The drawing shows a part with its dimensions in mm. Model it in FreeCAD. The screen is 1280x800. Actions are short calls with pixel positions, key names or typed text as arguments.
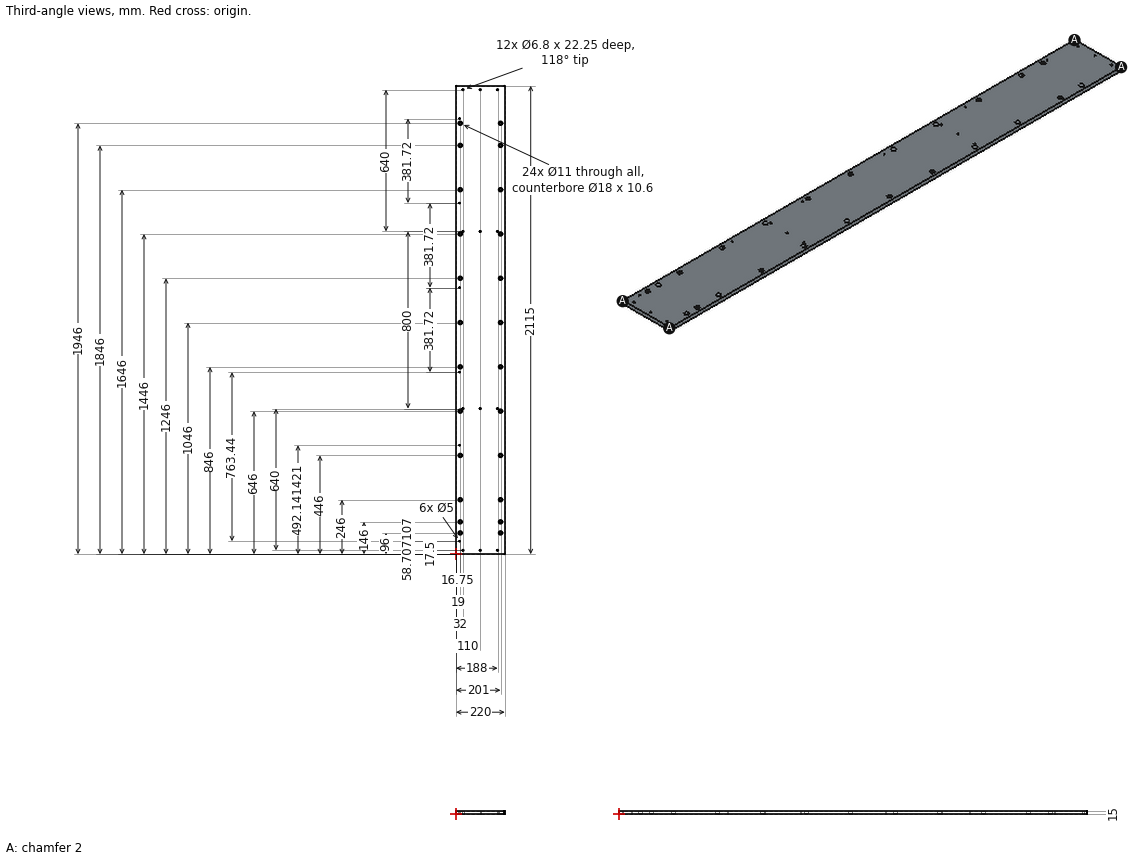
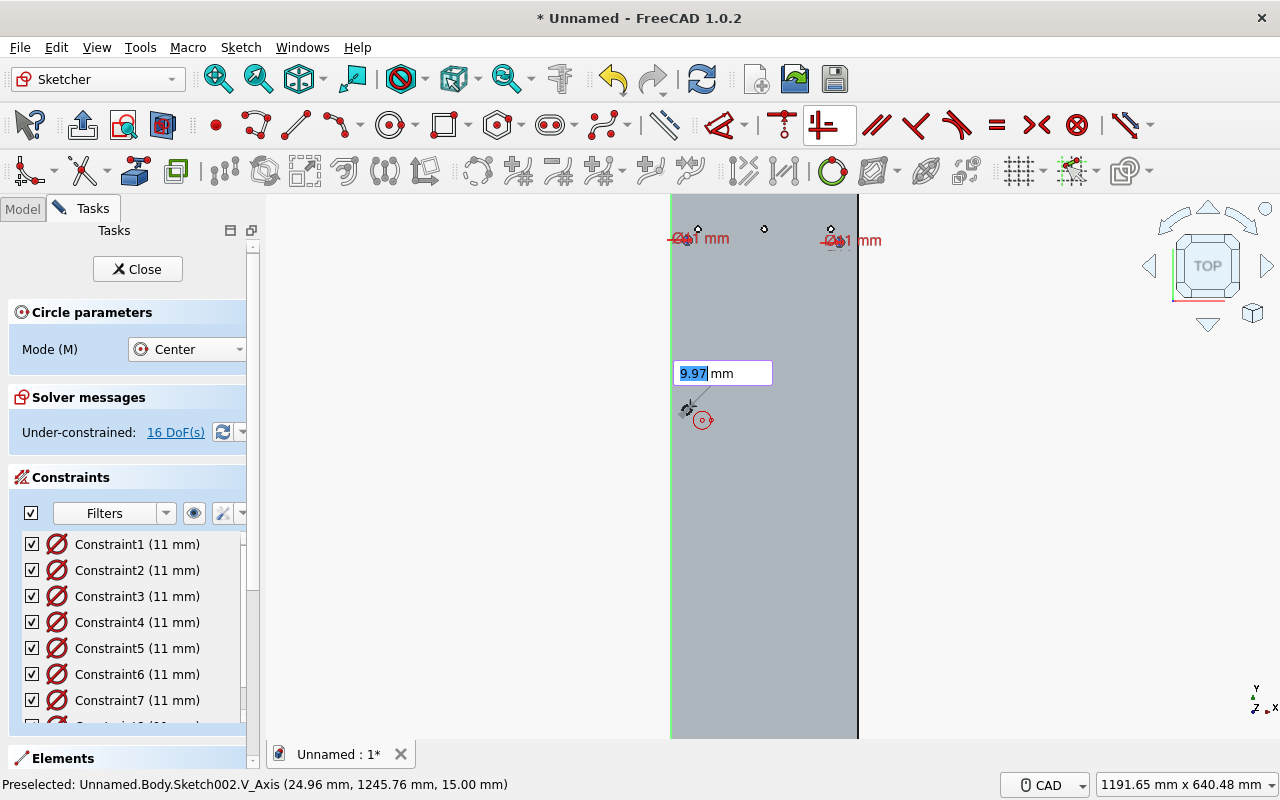
text(11)
key(Return)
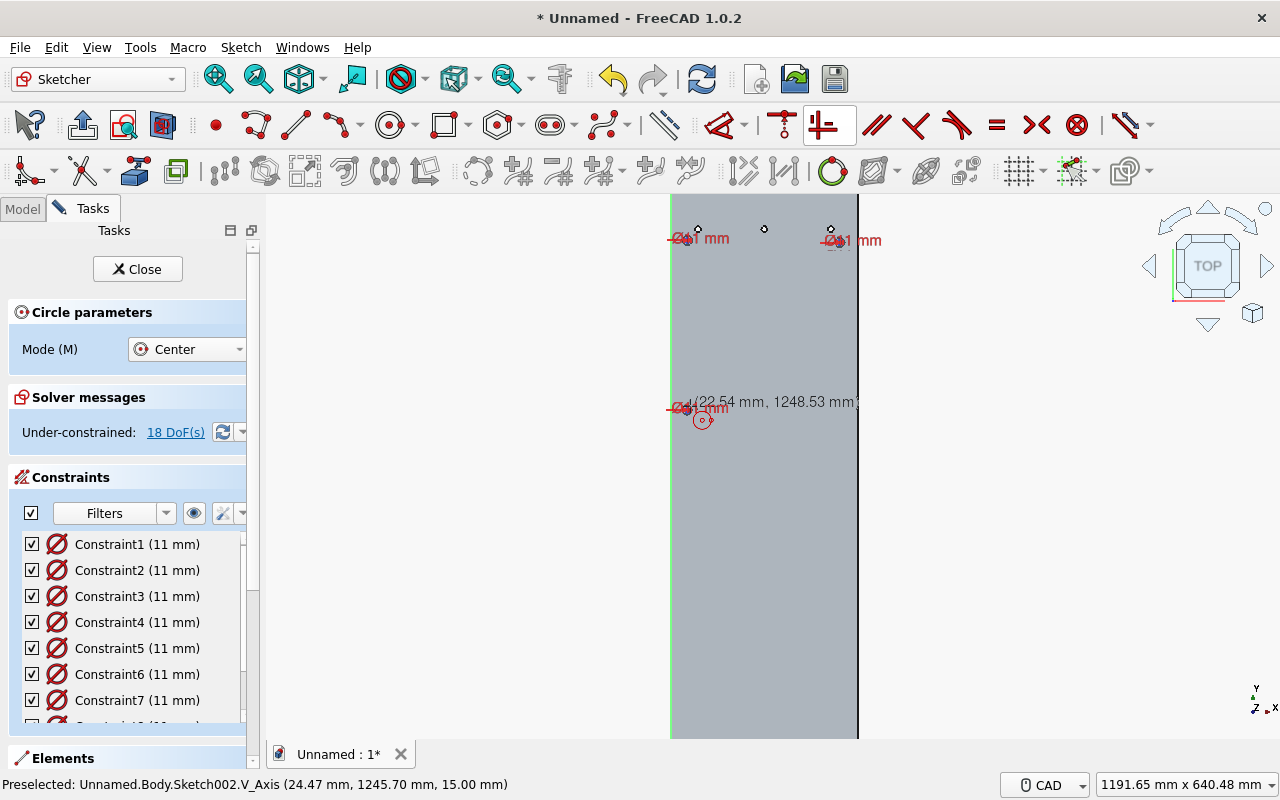
scroll(842, 409, up, 8)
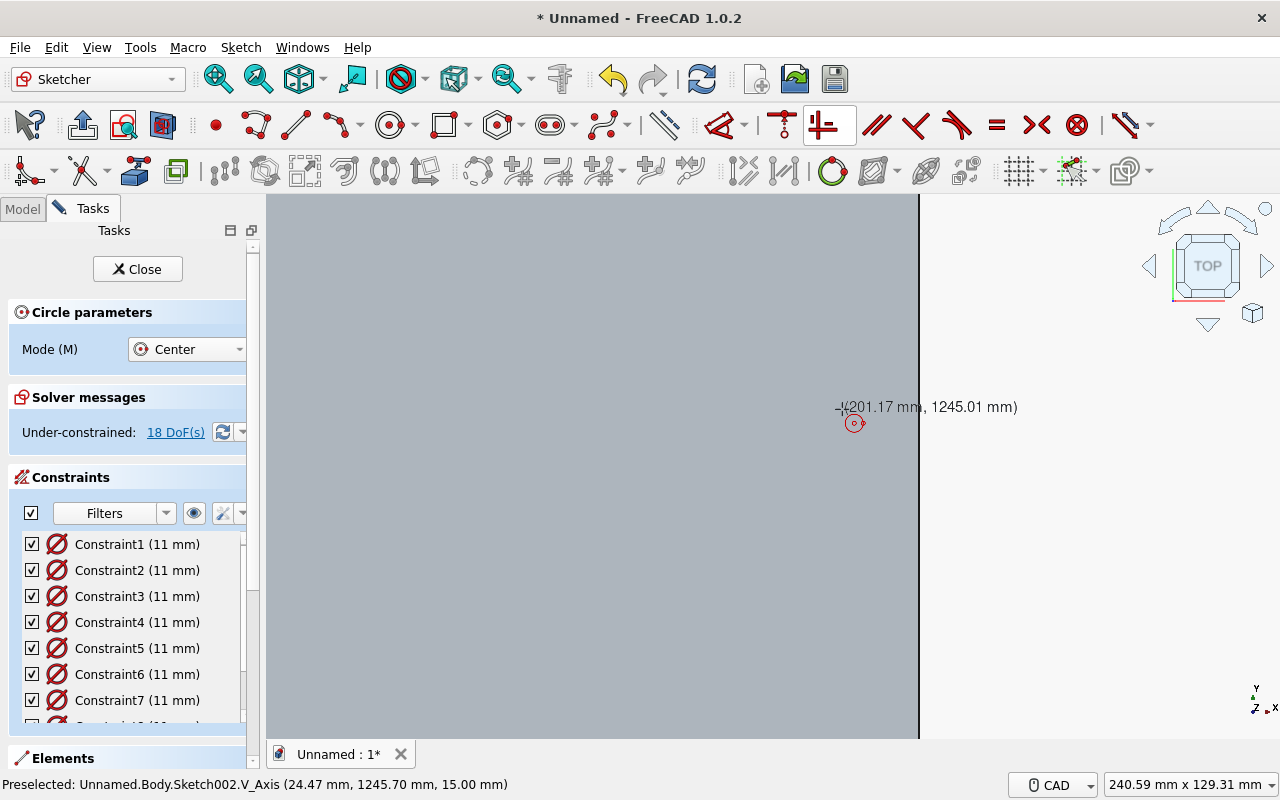
scroll(719, 410, down, 15)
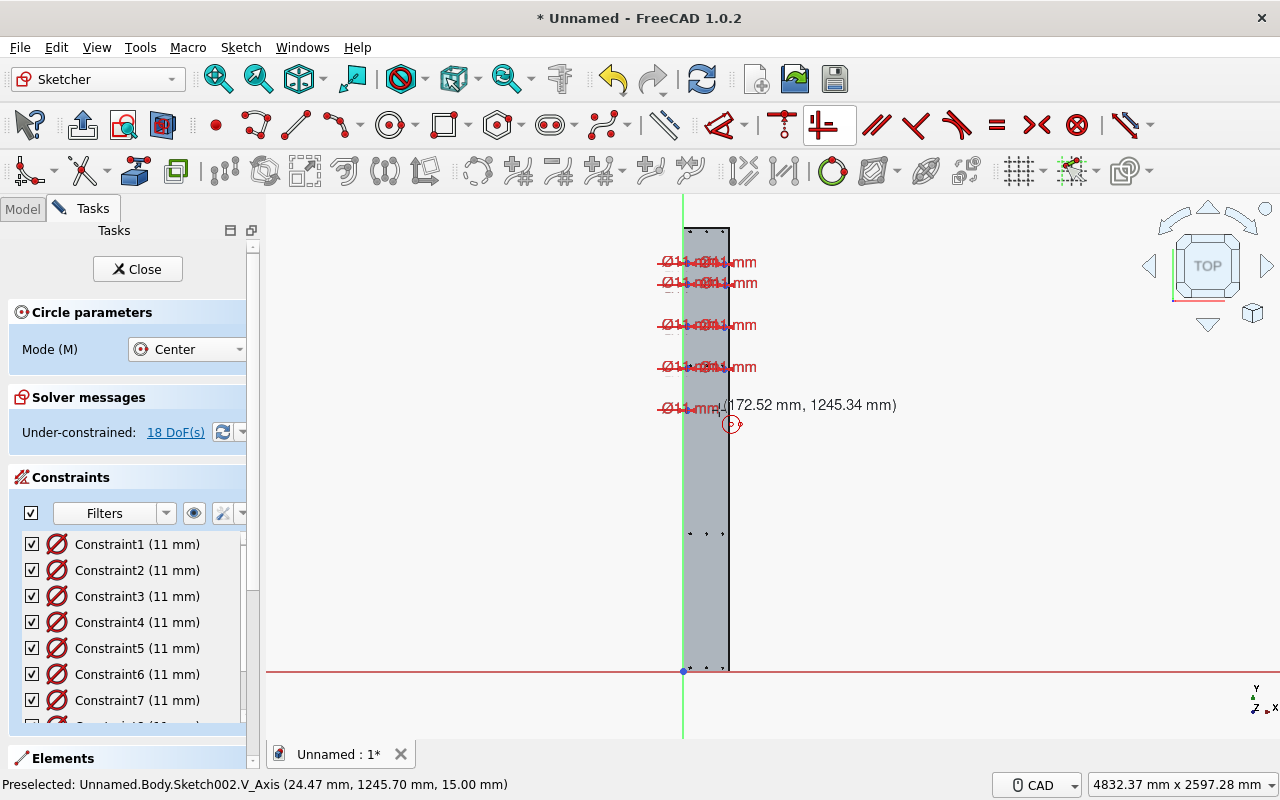
click(725, 410)
move(726, 409)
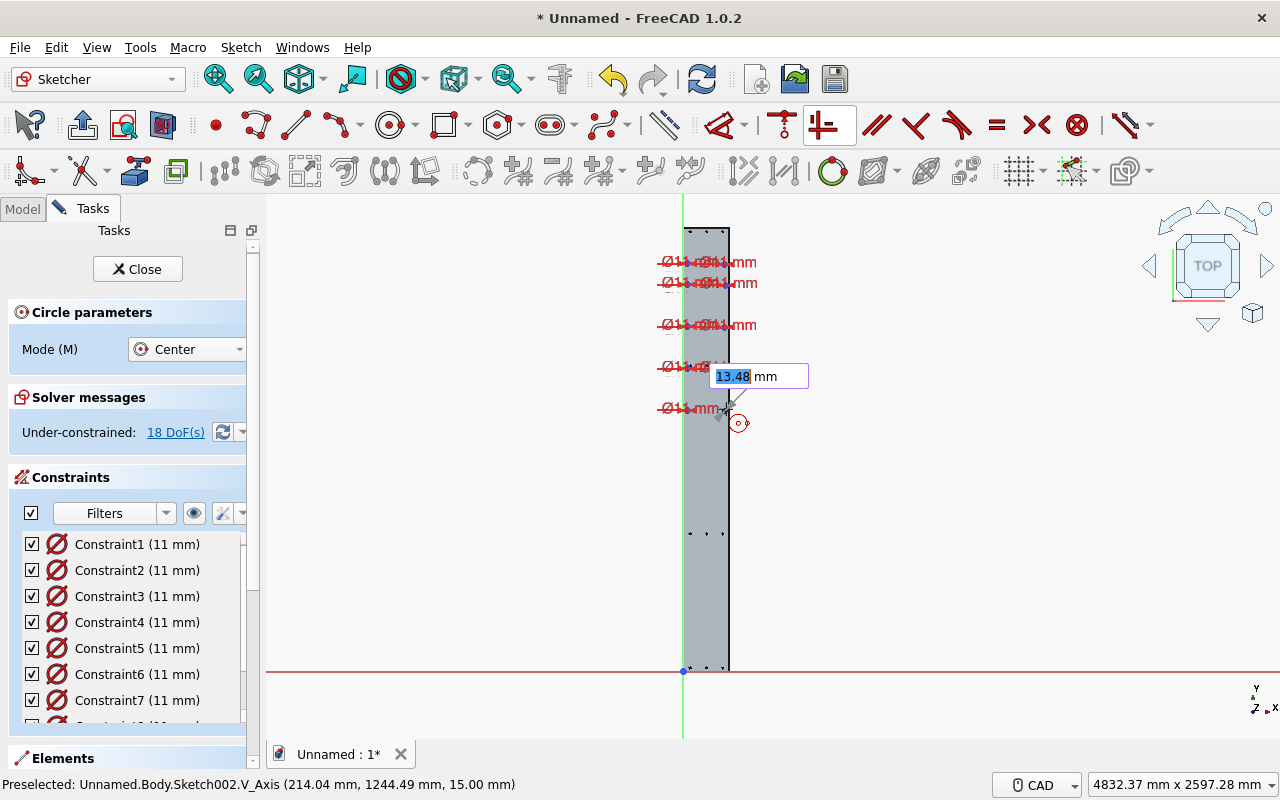
text(11)
key(Return)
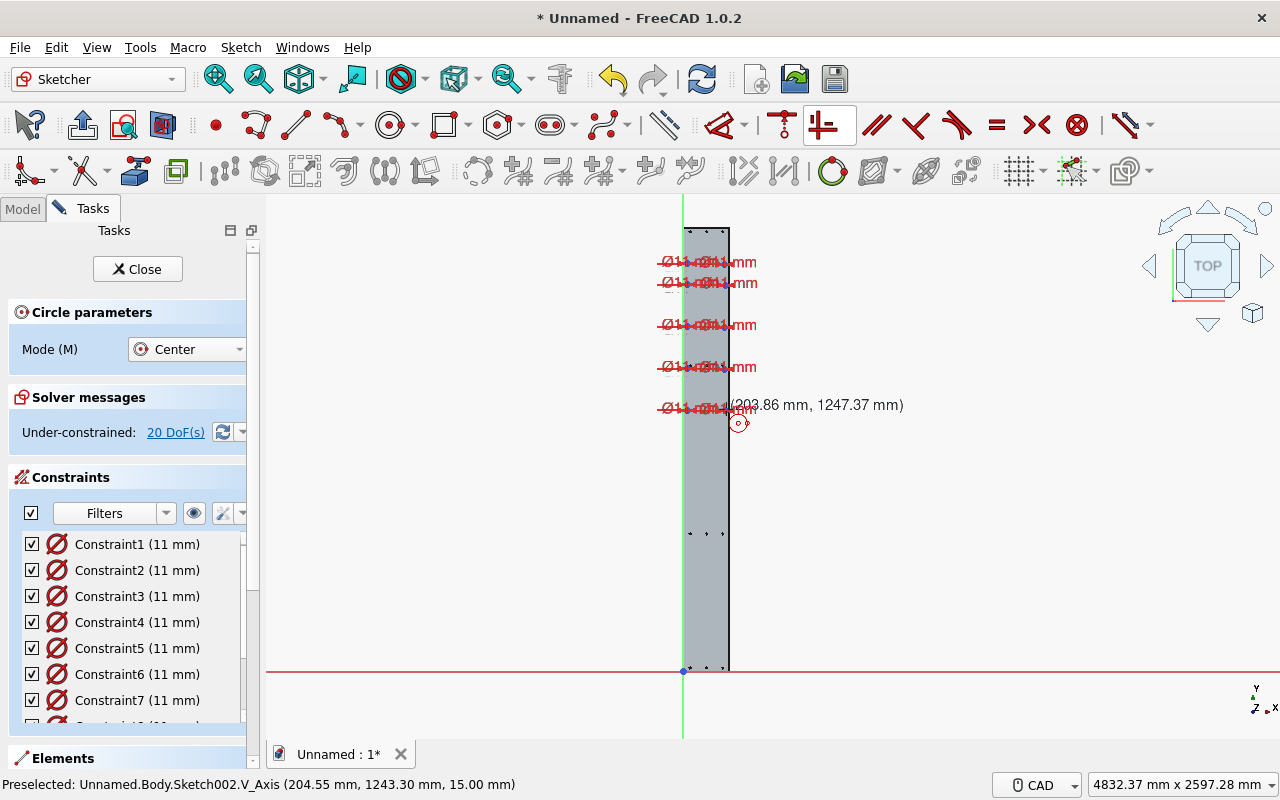
scroll(687, 452, up, 15)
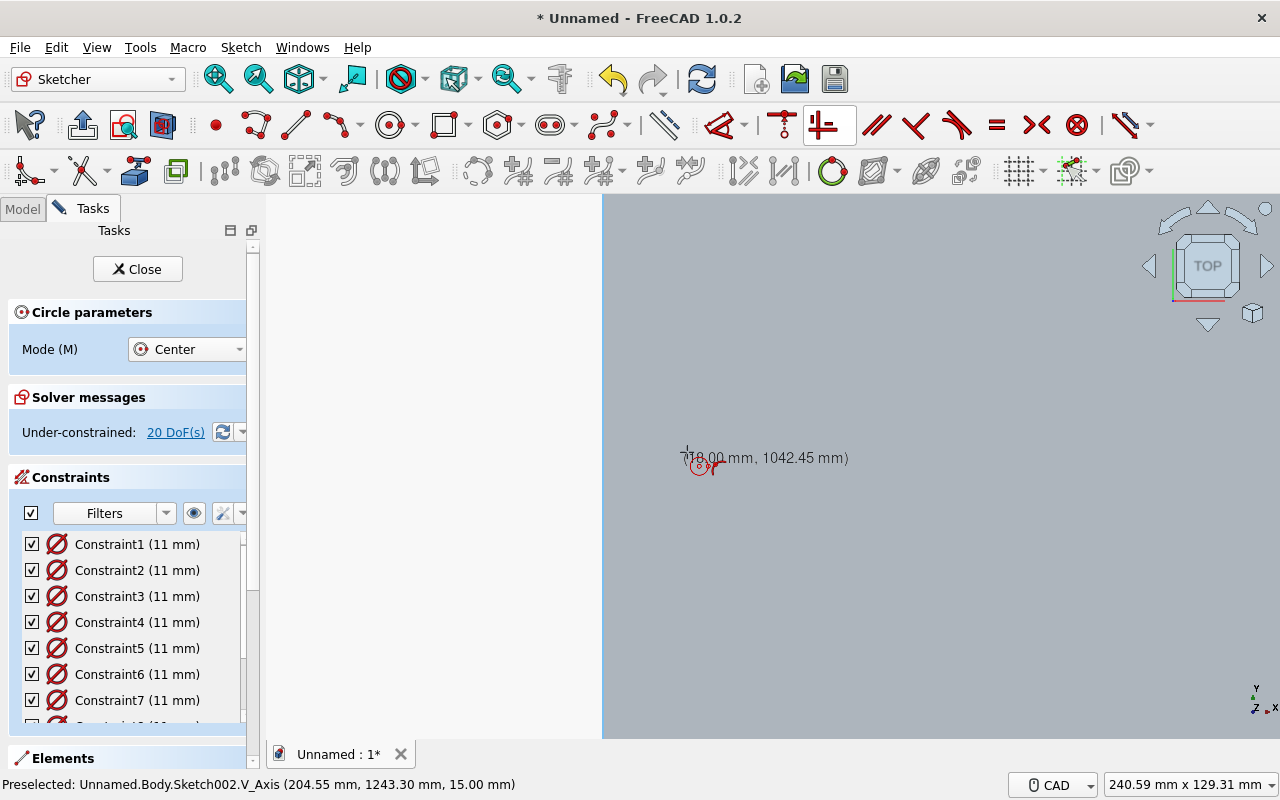
scroll(687, 452, down, 15)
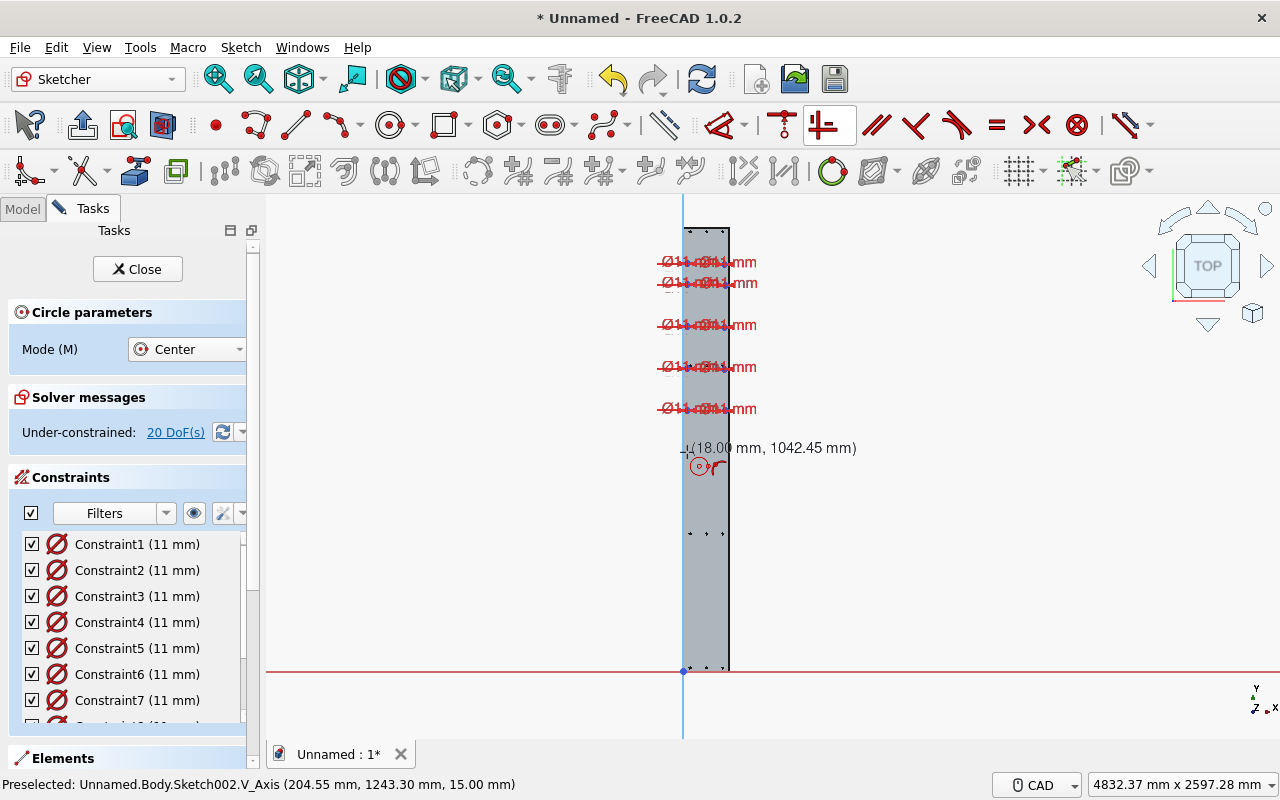
scroll(687, 452, up, 7)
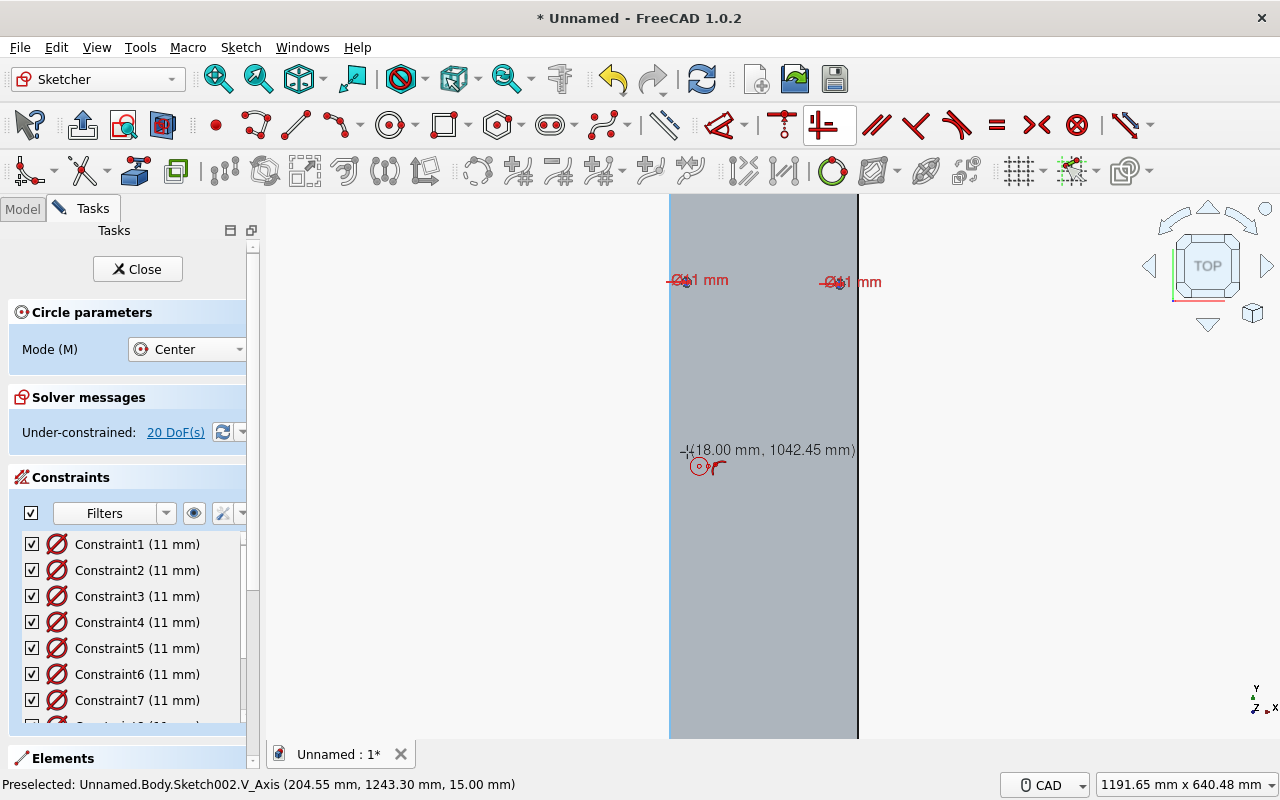
click(687, 452)
move(690, 448)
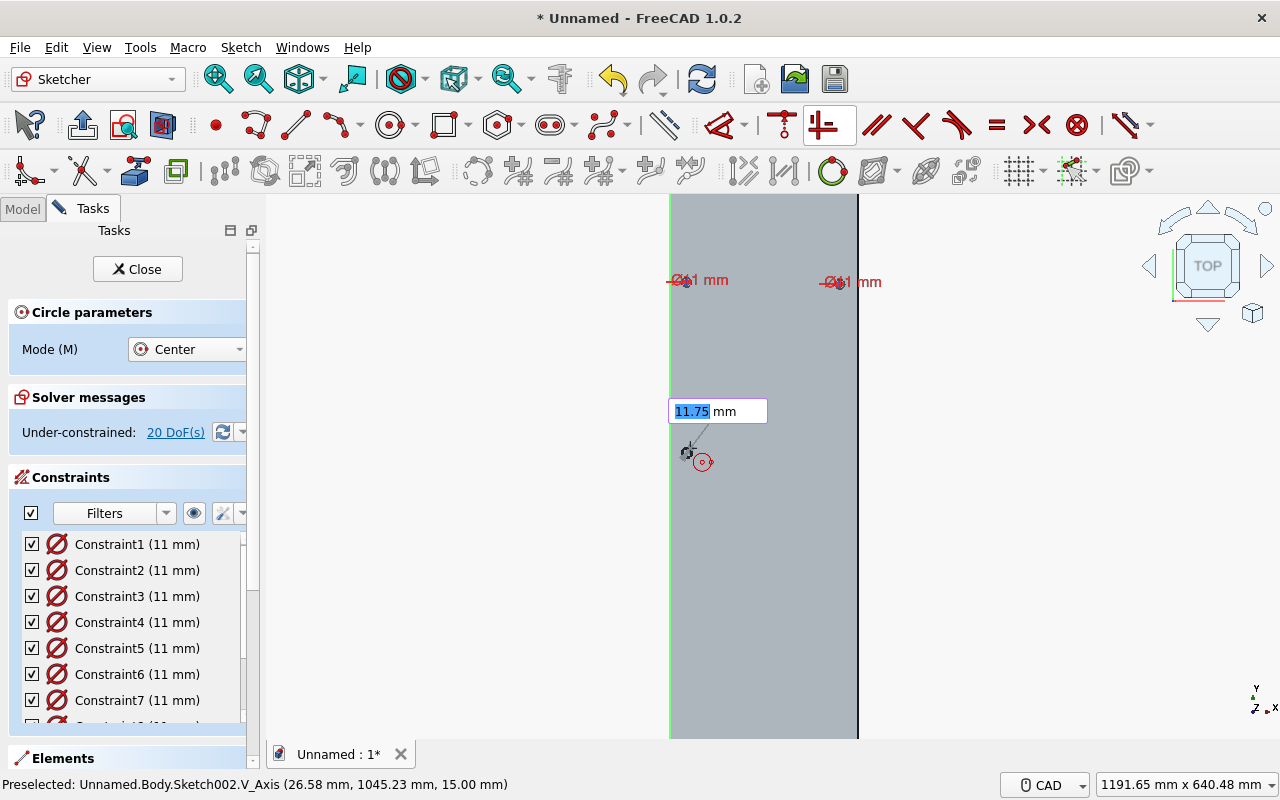
text(11)
key(Return)